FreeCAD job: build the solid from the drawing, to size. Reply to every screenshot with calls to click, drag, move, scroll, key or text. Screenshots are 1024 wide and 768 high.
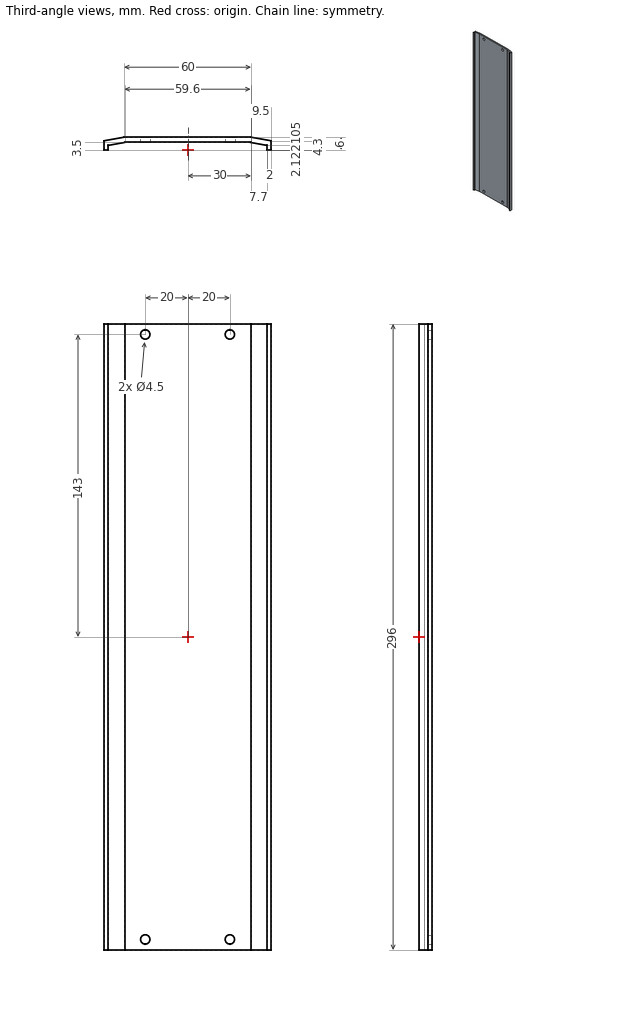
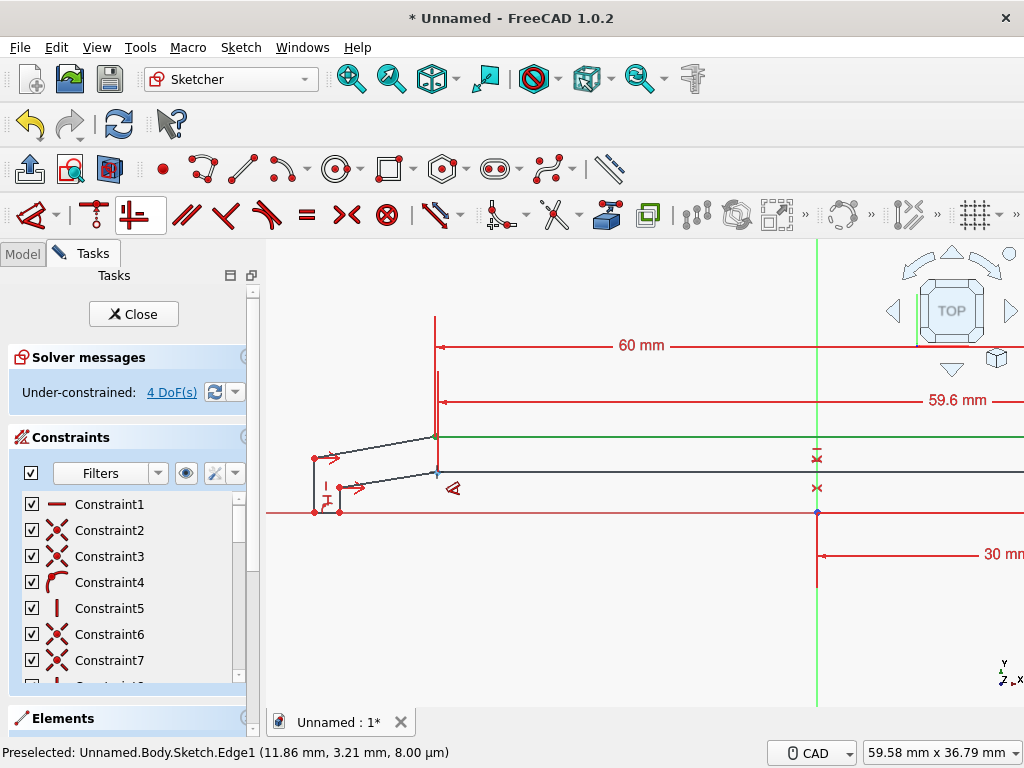
click(438, 472)
click(404, 492)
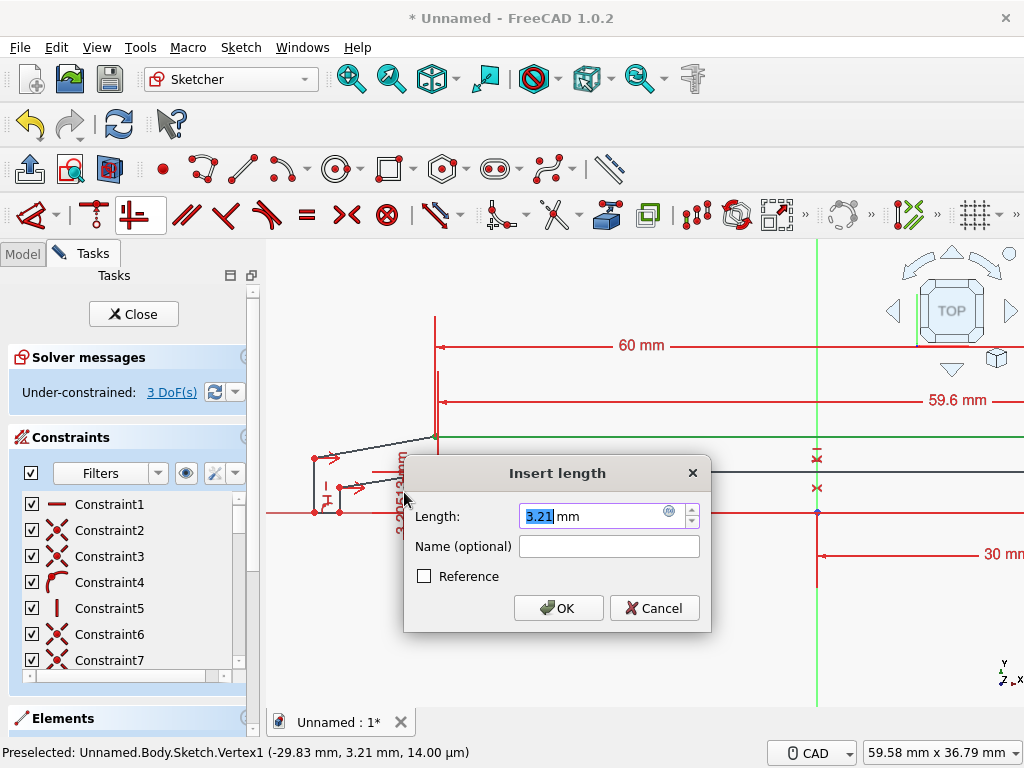
text(3.5)
key(Return)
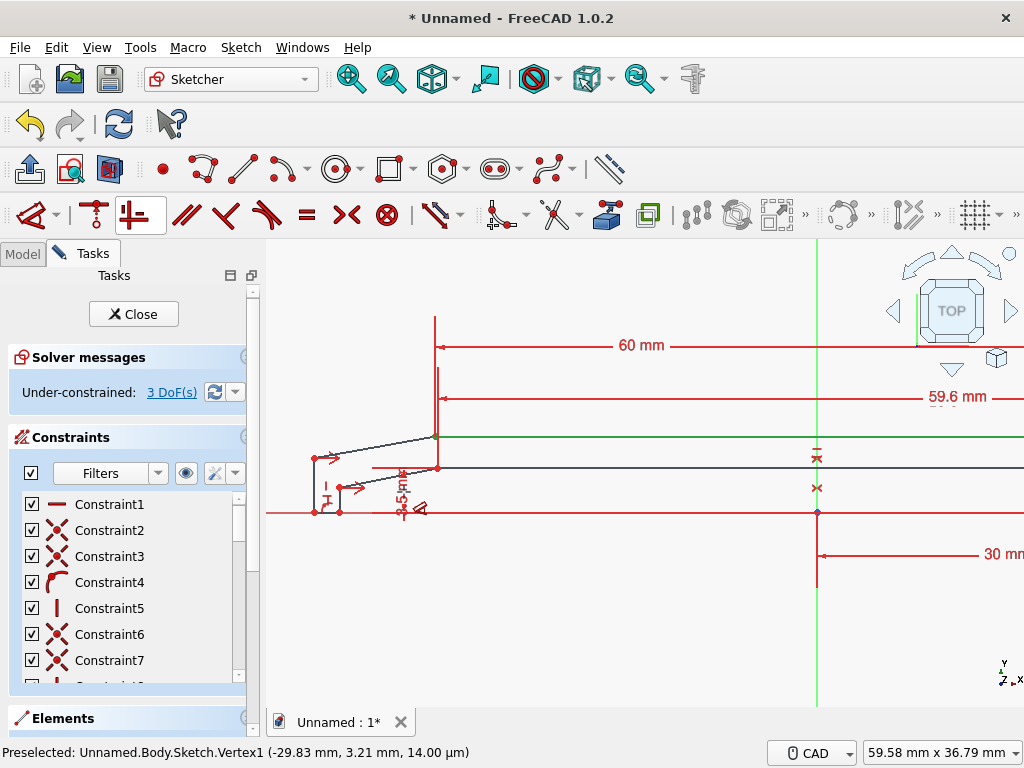
scroll(436, 472, down, 5)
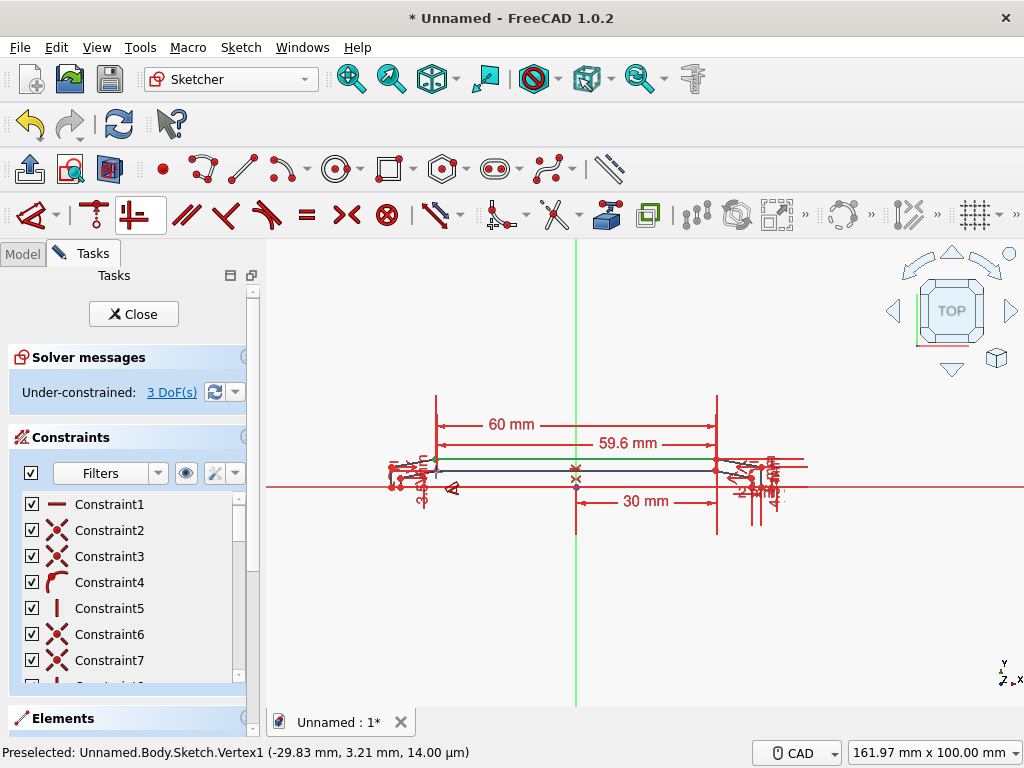
scroll(727, 473, up, 2)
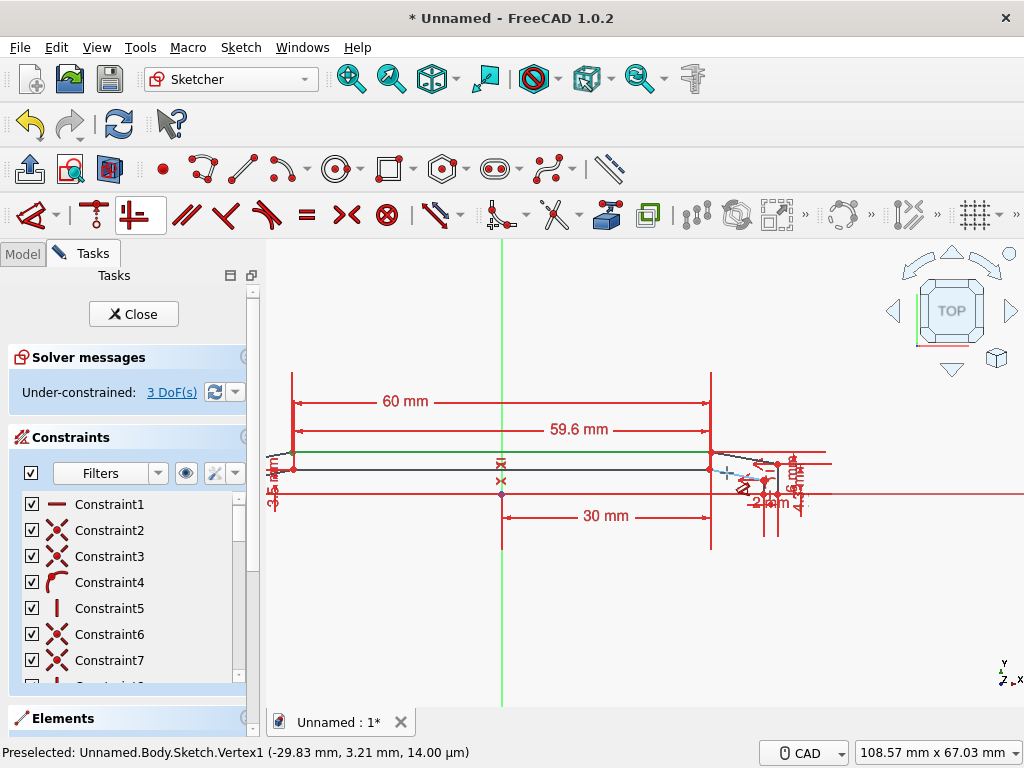
click(726, 473)
click(737, 436)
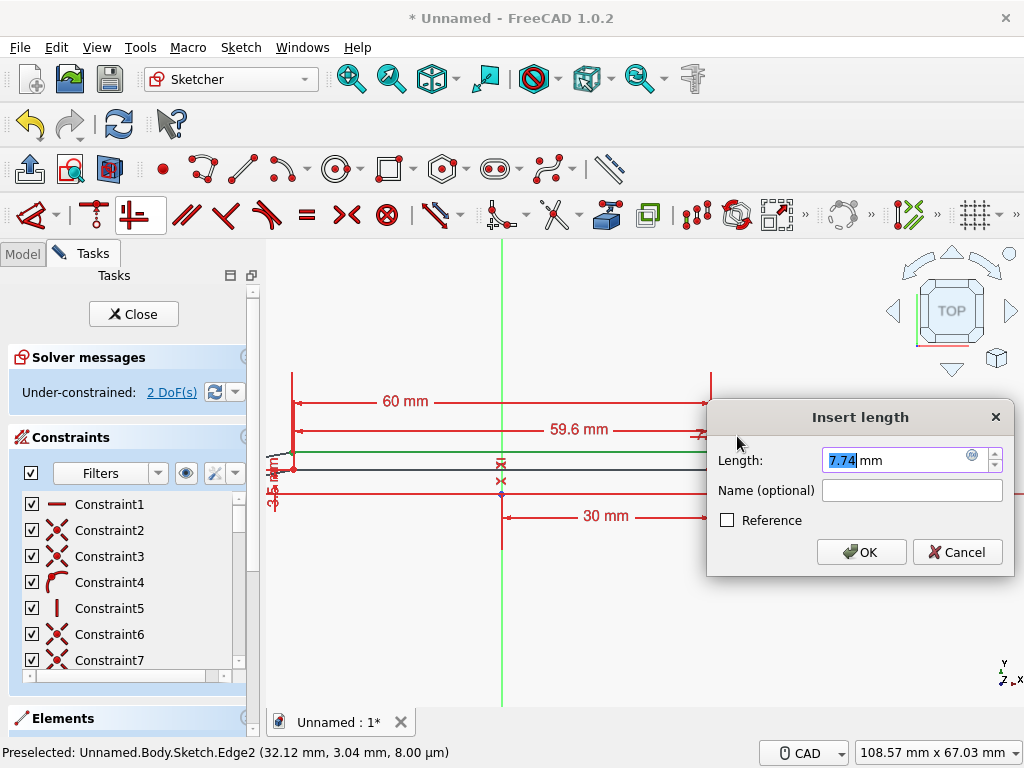
text(7.7)
key(Return)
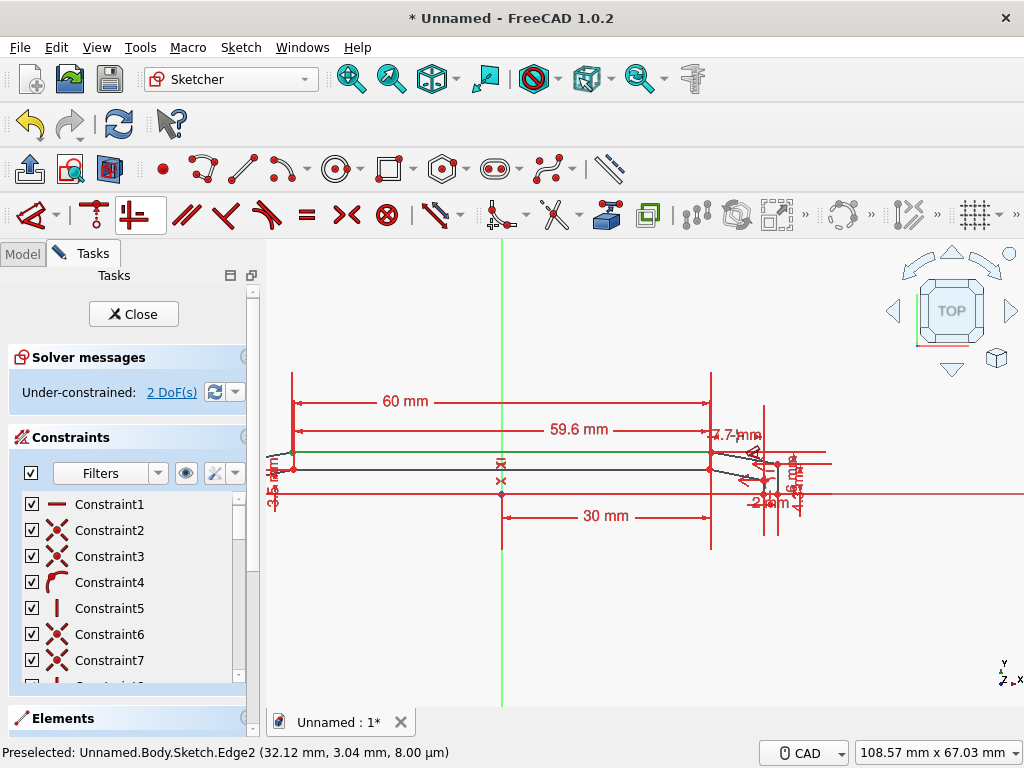
click(758, 461)
click(744, 394)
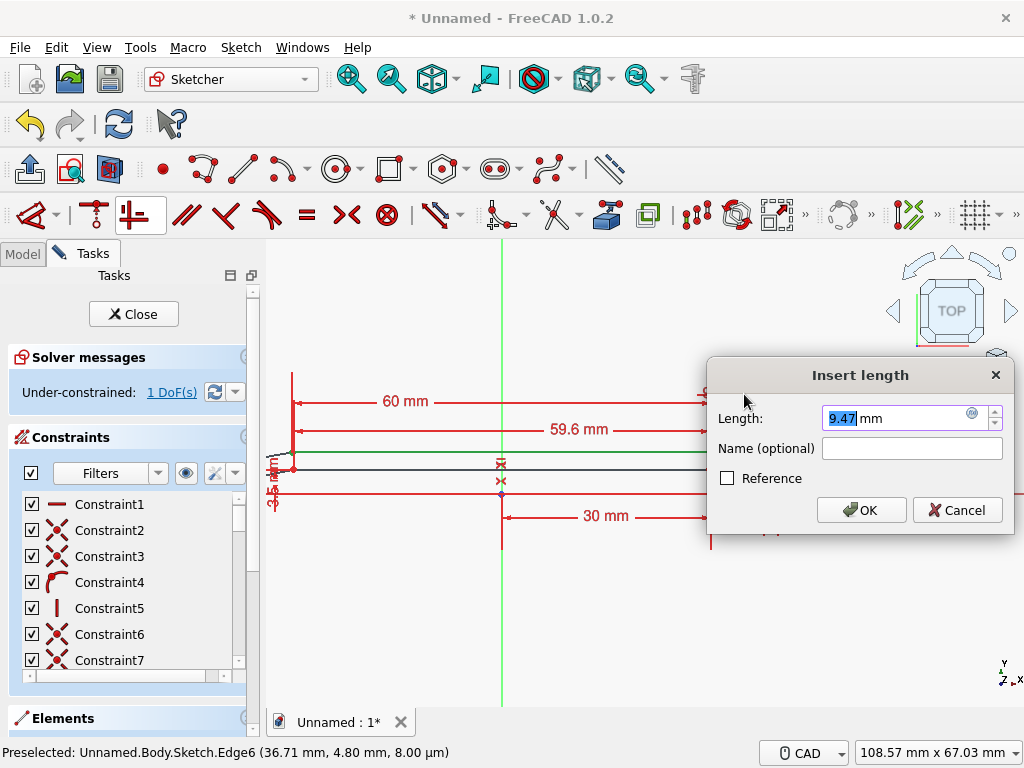
text(9.5)
key(Return)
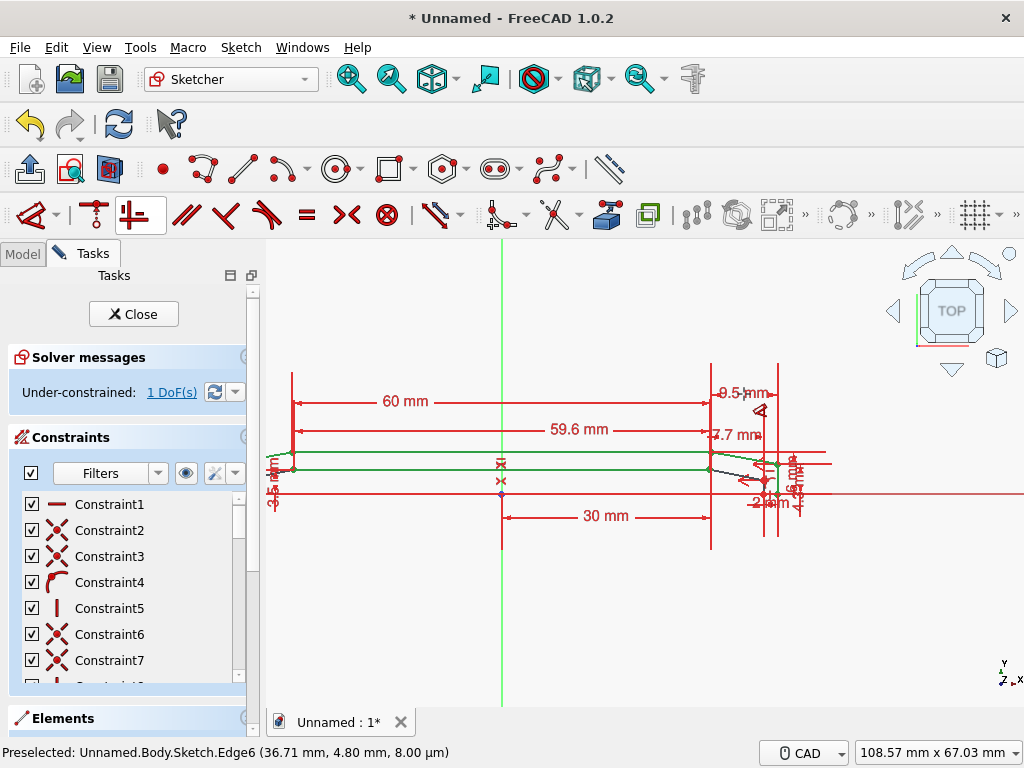
scroll(764, 487, up, 5)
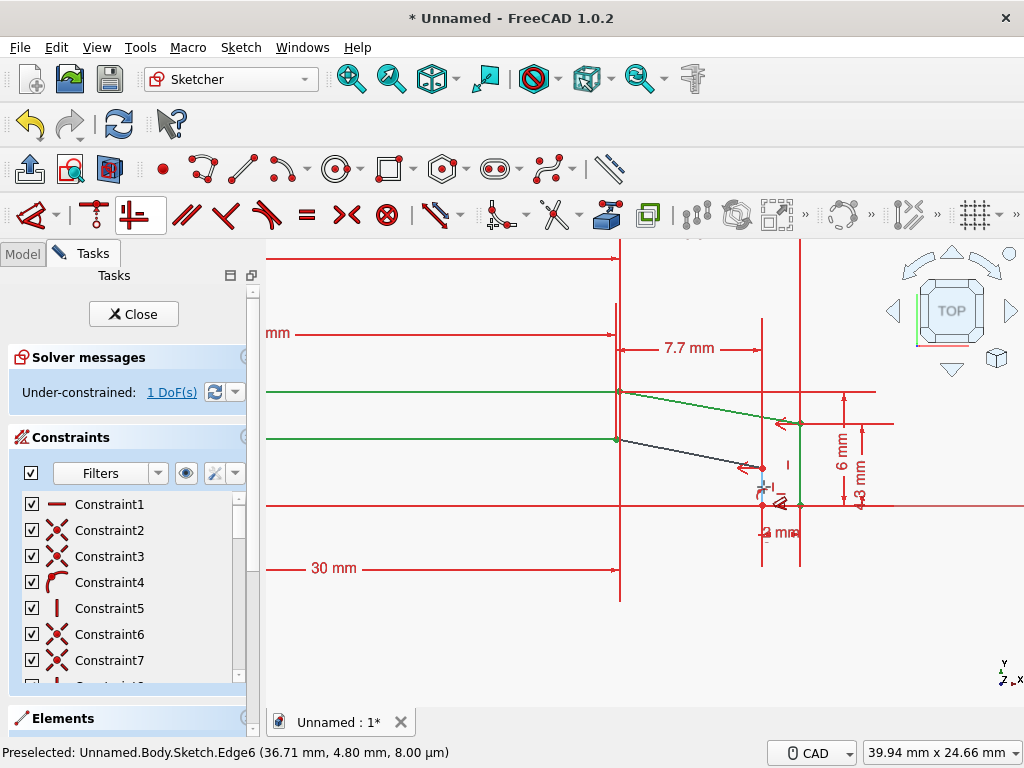
click(762, 487)
click(728, 487)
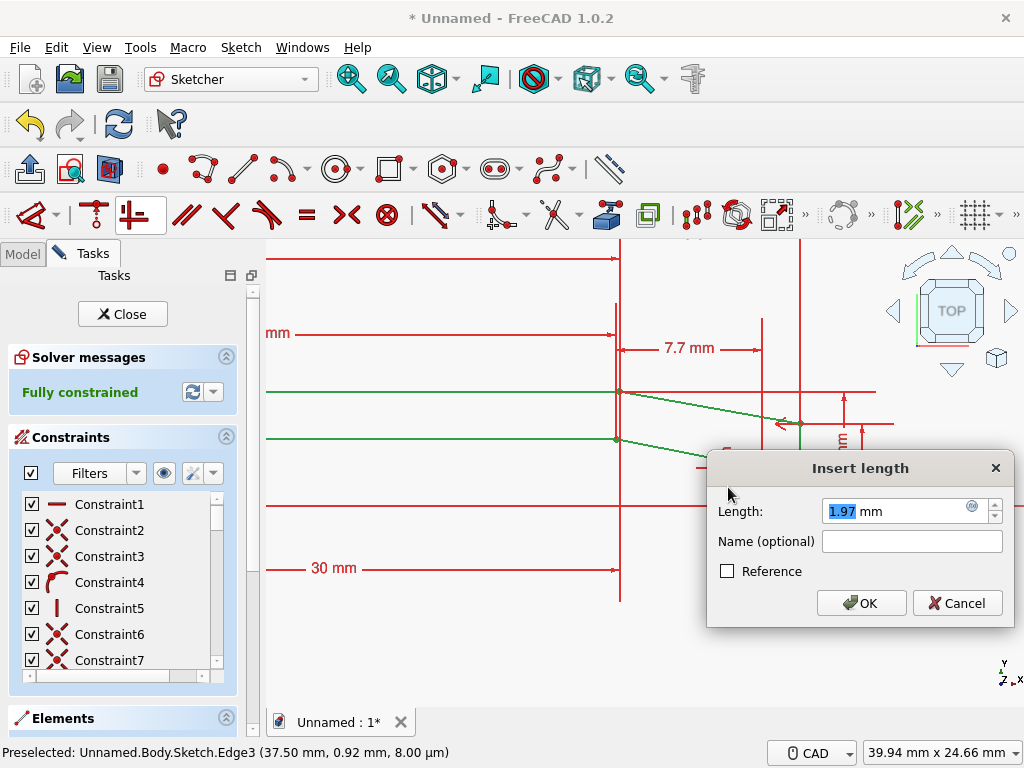
text(2.122105)
key(Return)
key(Escape)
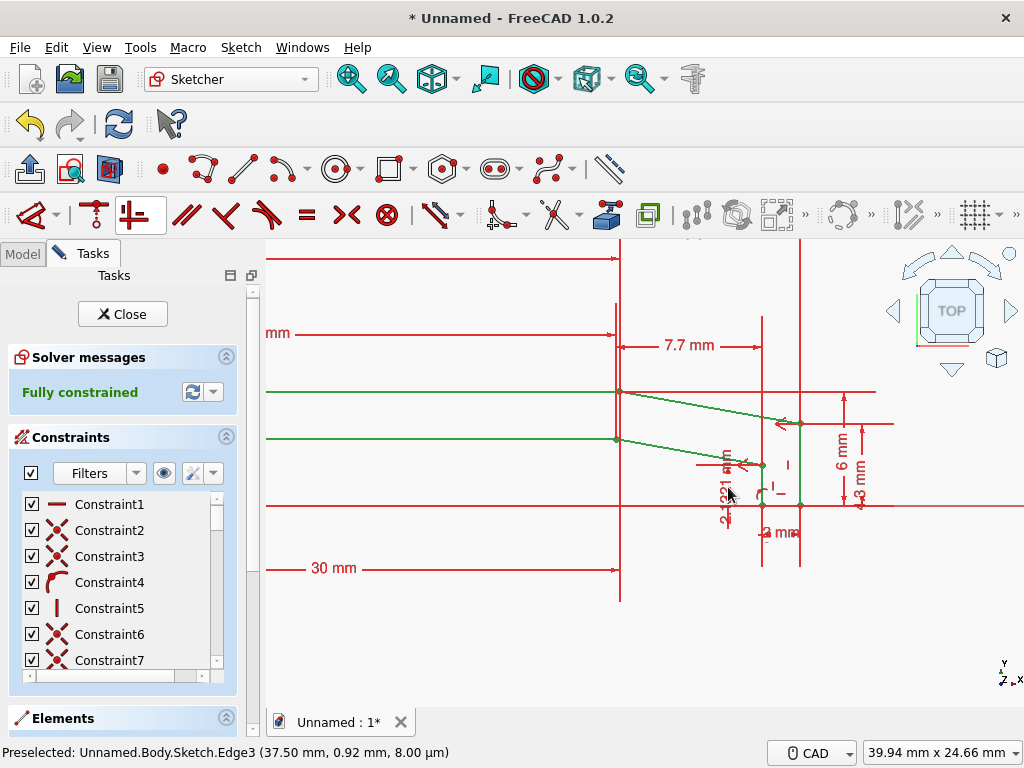
click(123, 314)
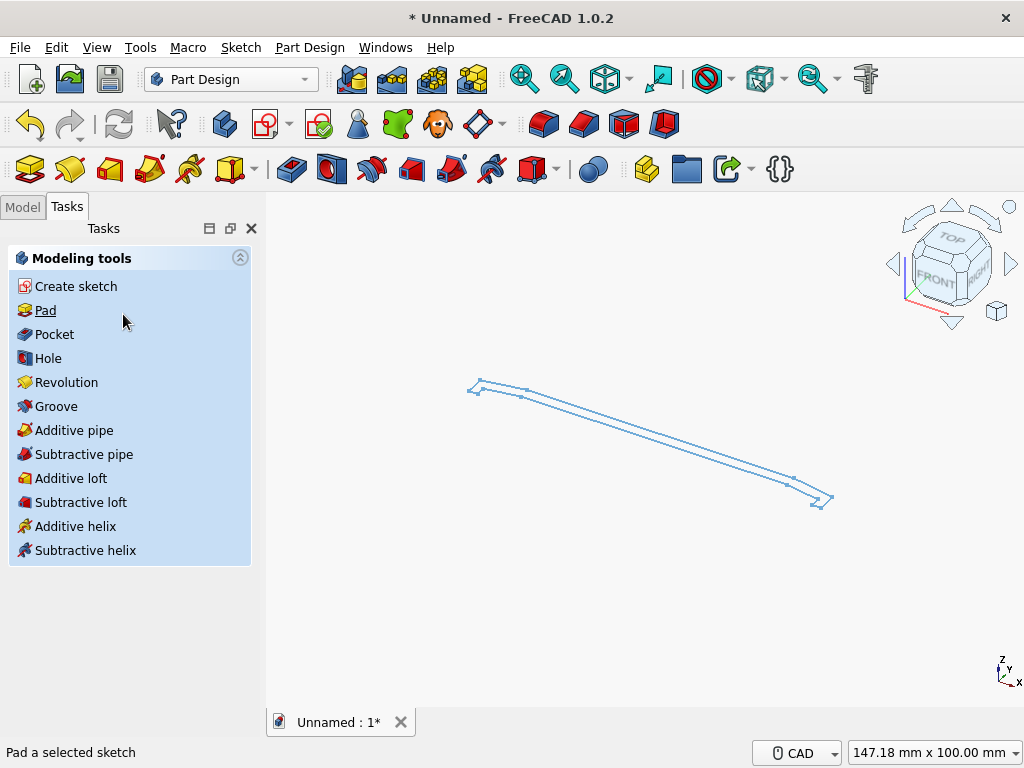
click(30, 170)